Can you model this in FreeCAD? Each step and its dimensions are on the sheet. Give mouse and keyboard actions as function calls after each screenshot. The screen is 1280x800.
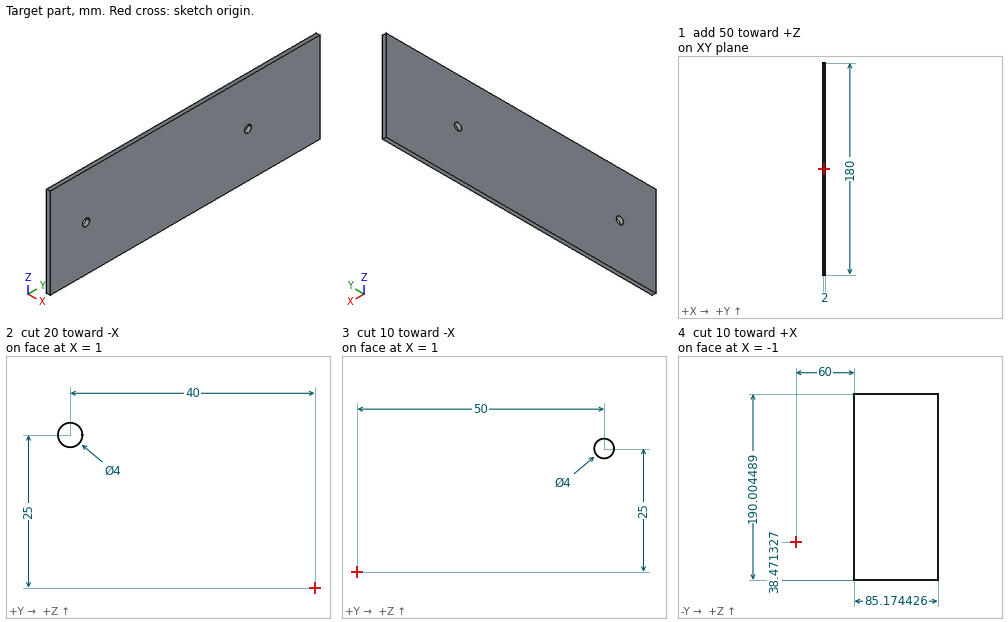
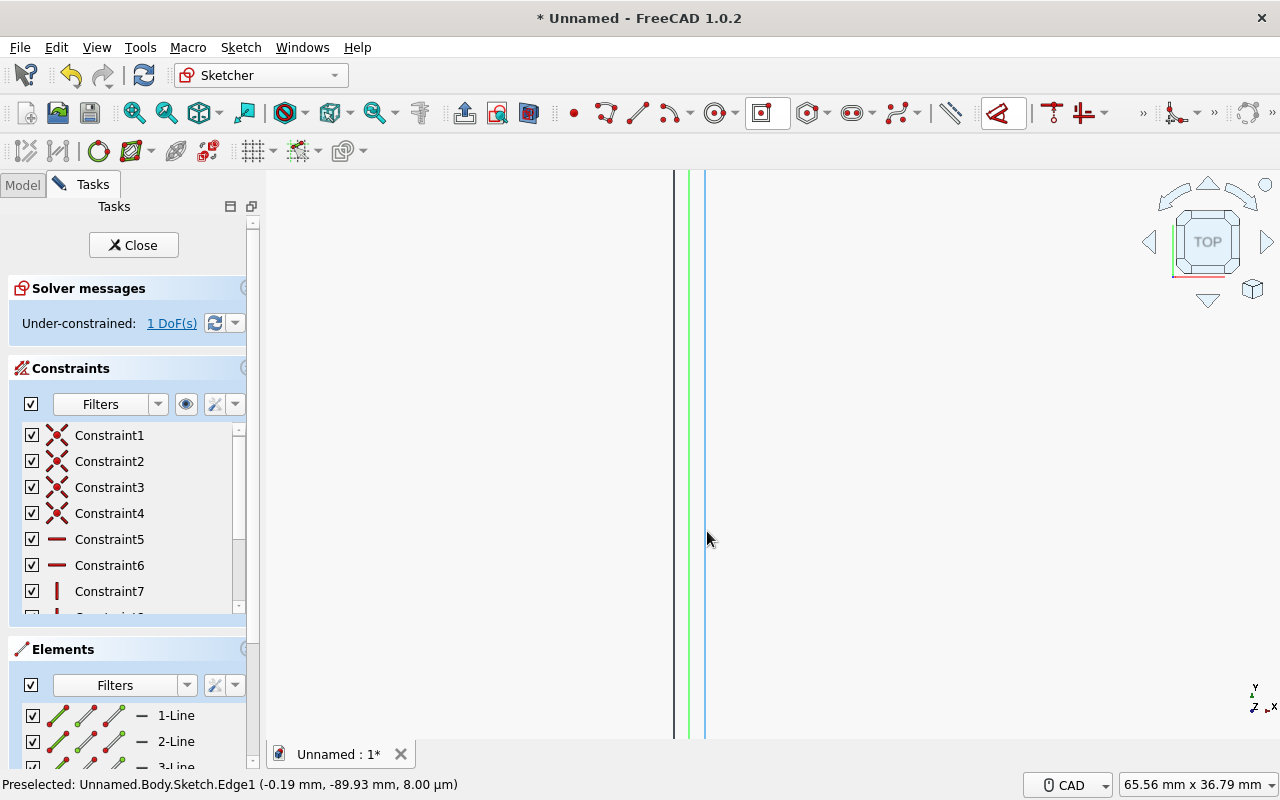
click(705, 525)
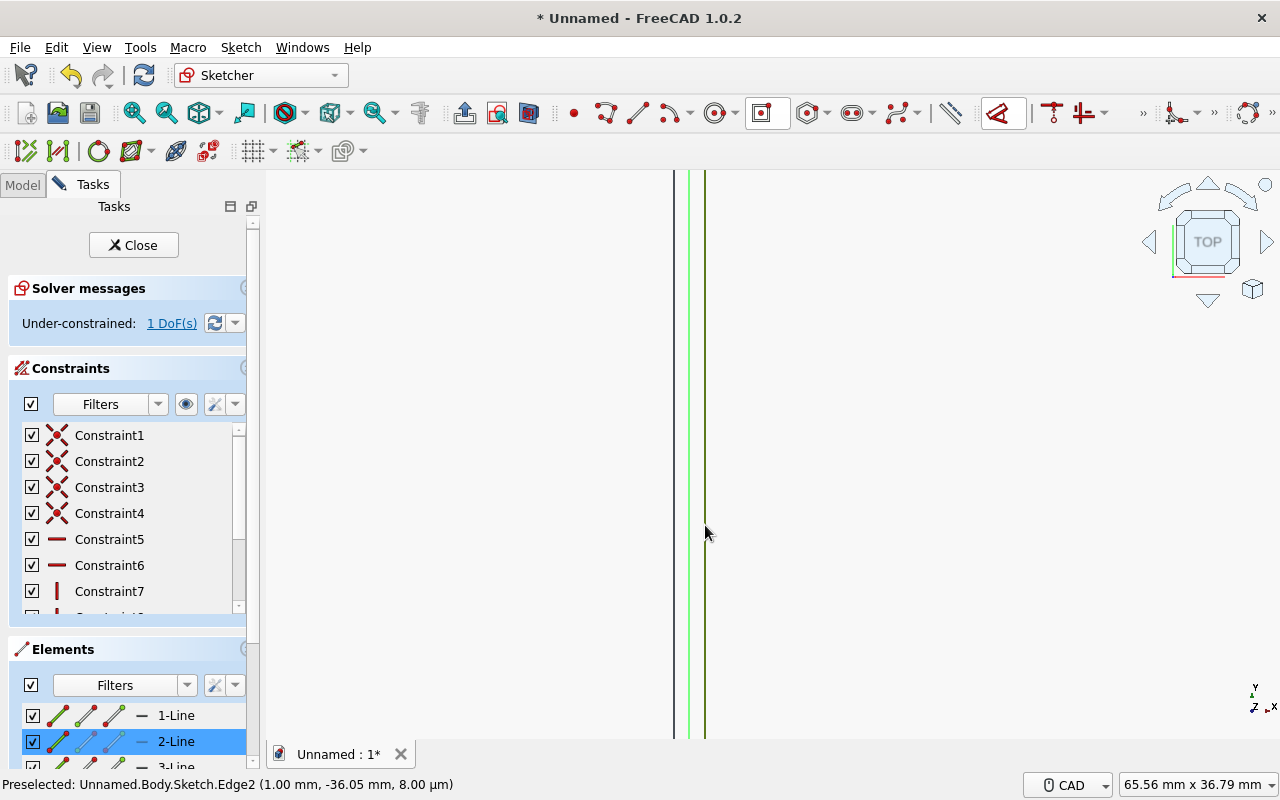
key(i)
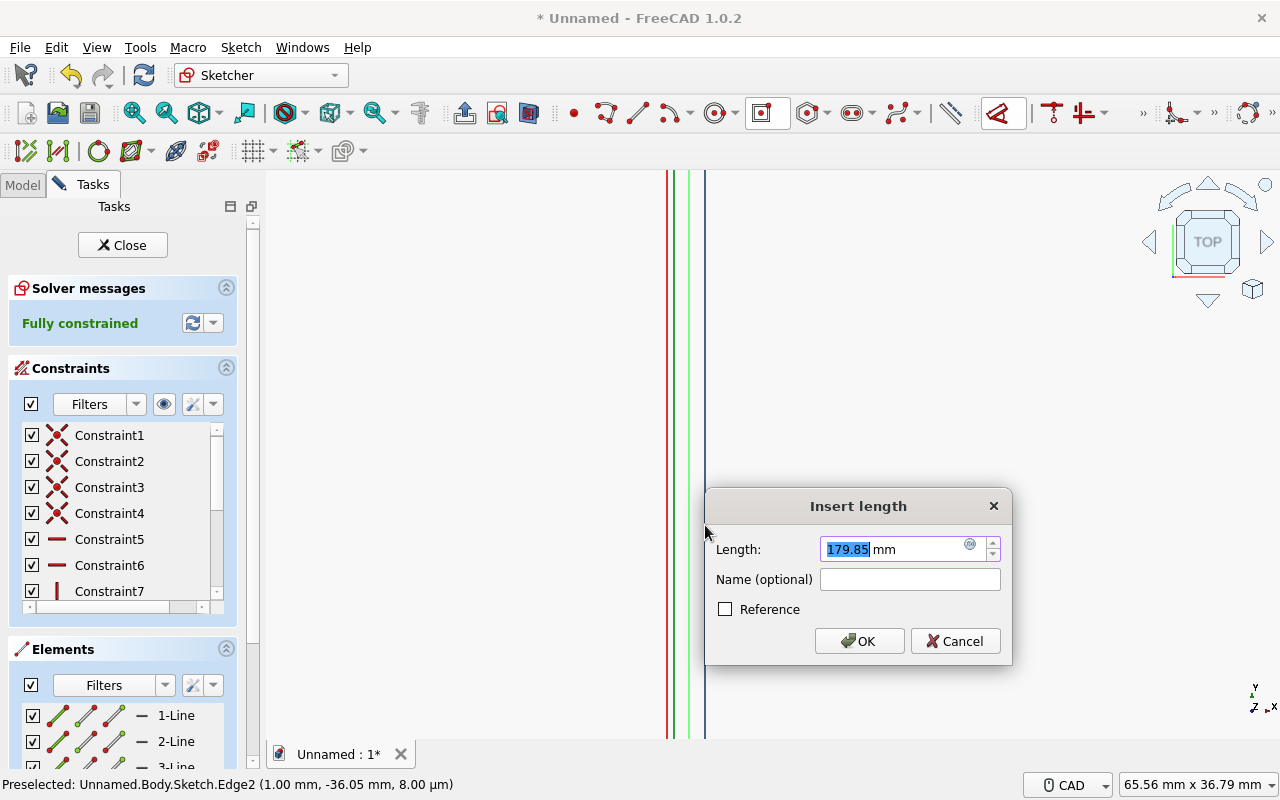
text(180)
key(Return)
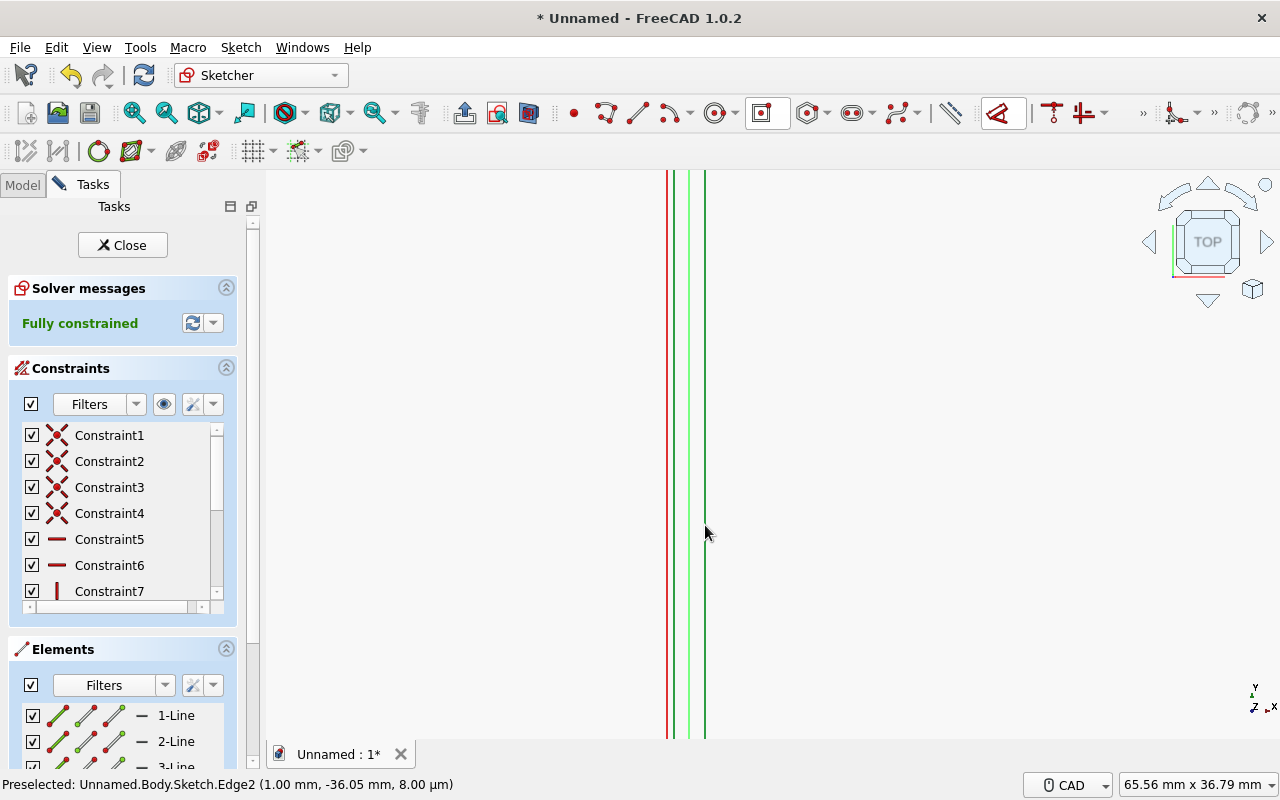
click(123, 245)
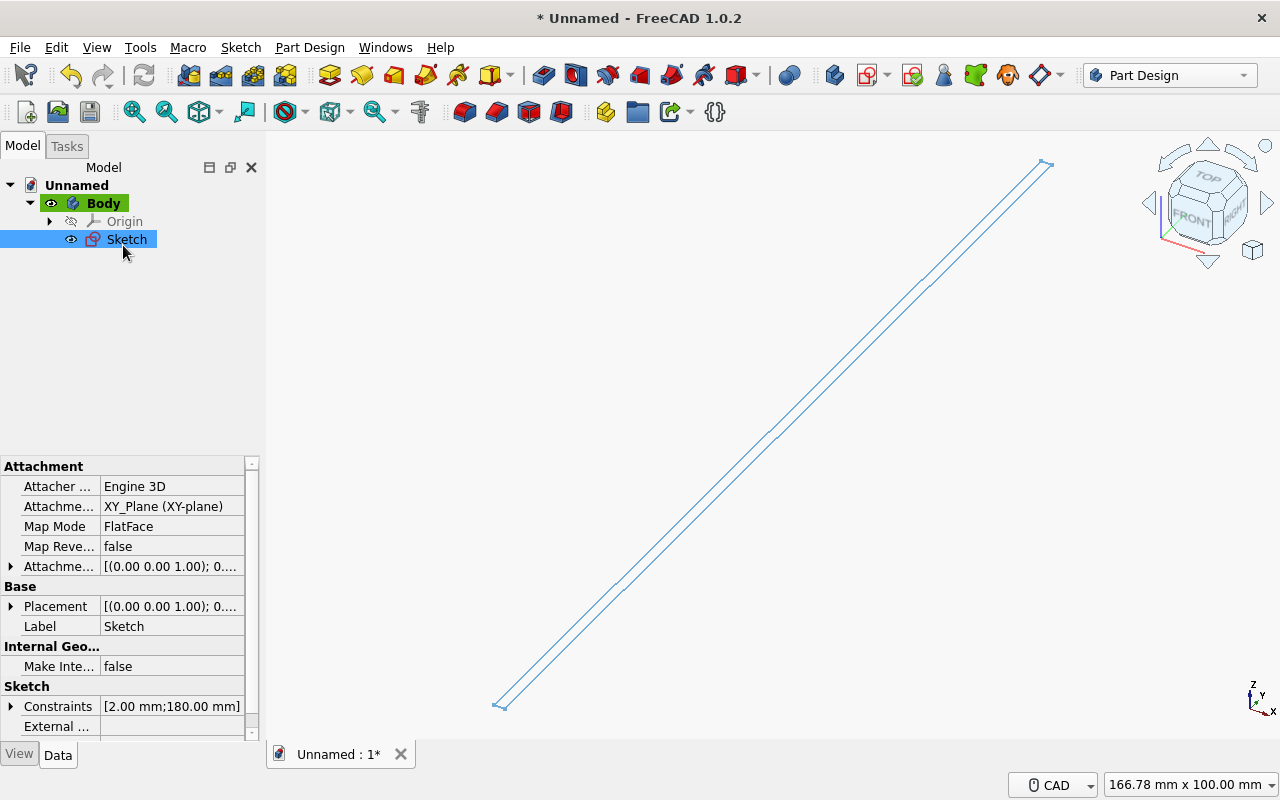
click(330, 76)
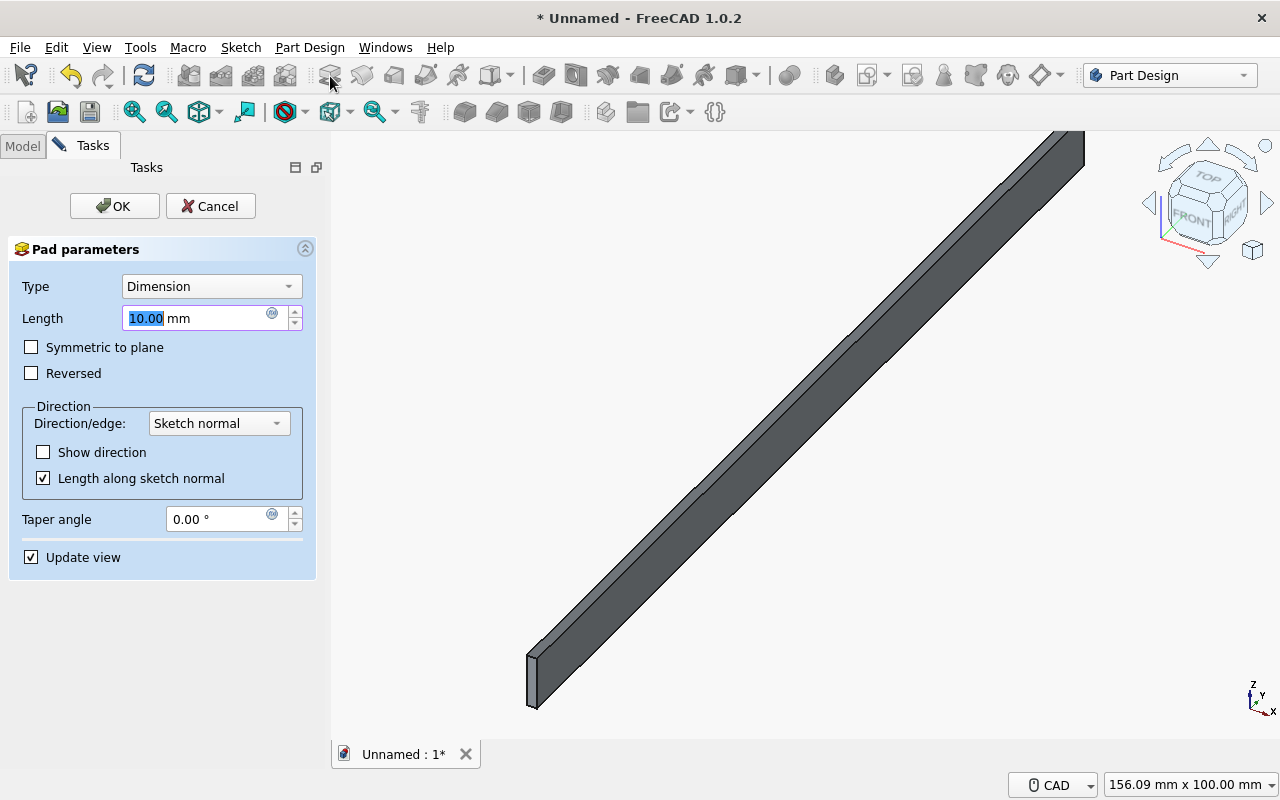
text(50)
key(Tab)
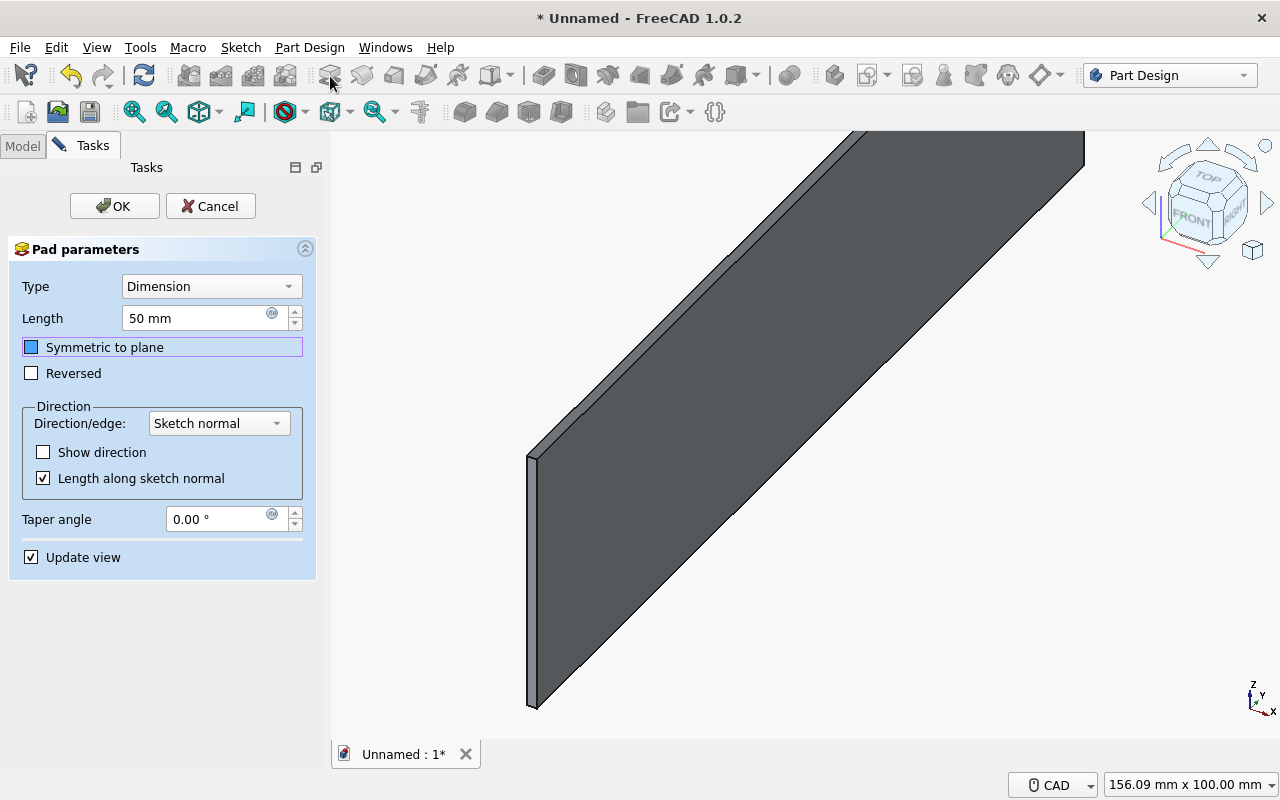
click(115, 206)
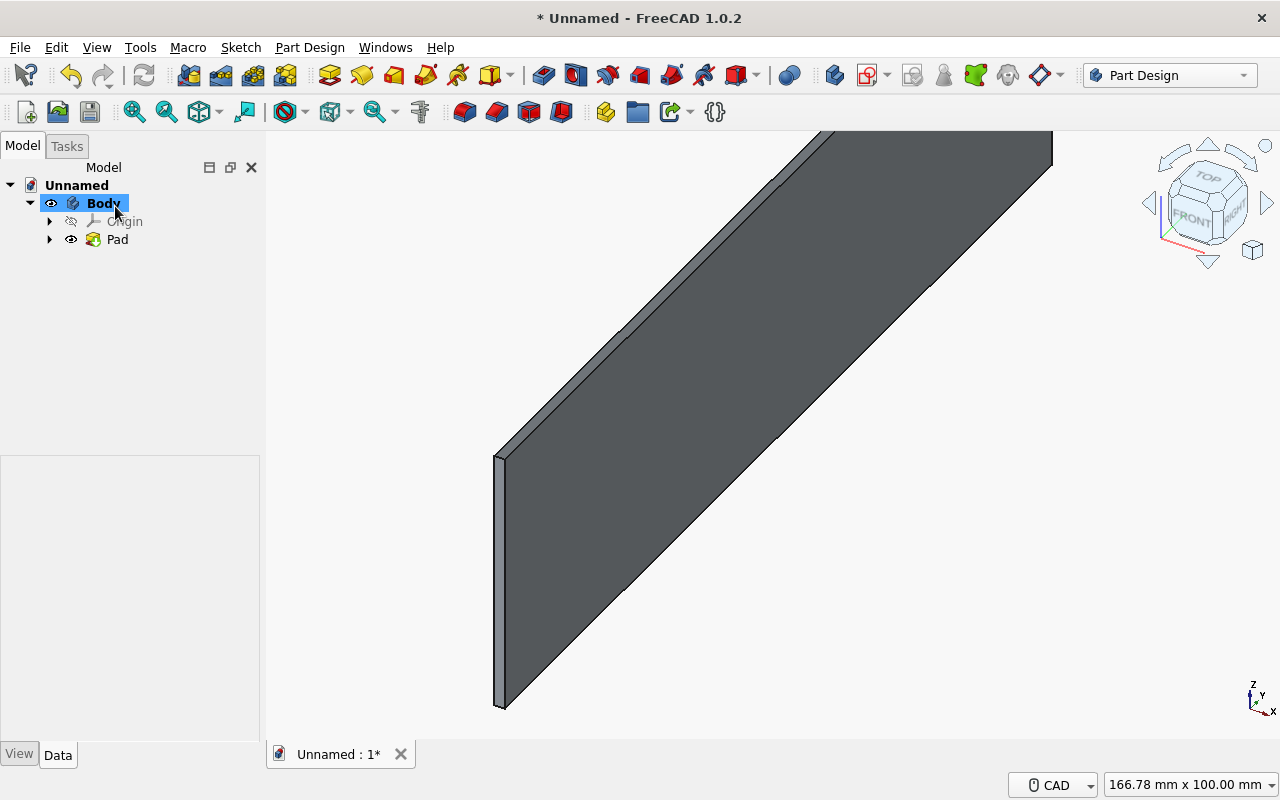
click(136, 112)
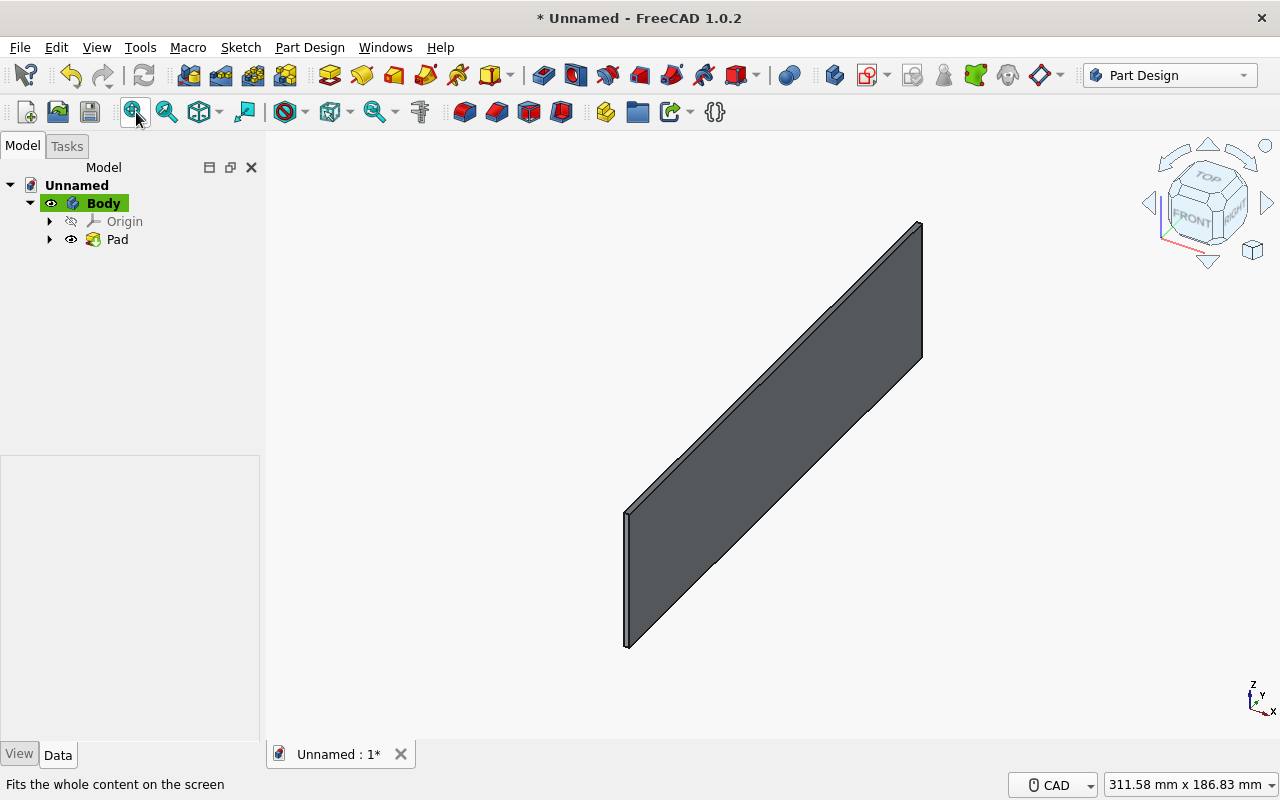
click(860, 352)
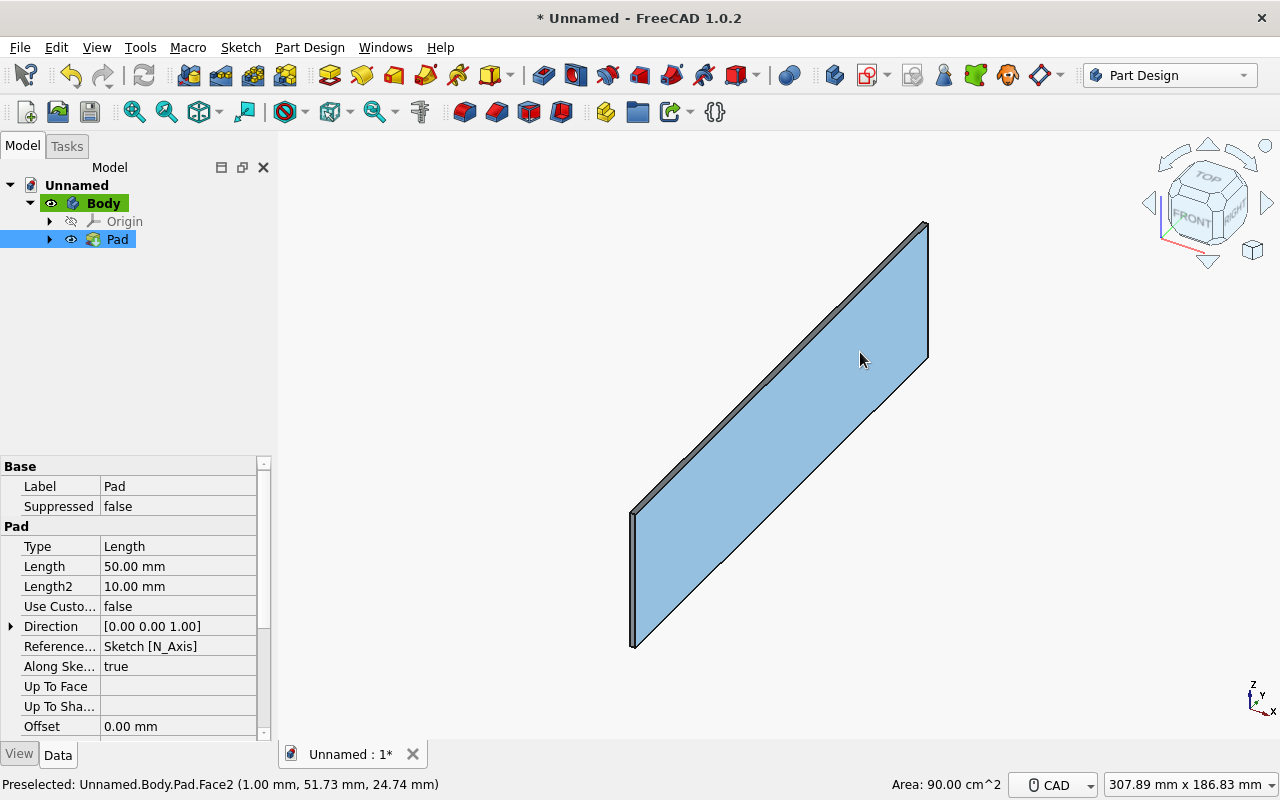
click(868, 76)